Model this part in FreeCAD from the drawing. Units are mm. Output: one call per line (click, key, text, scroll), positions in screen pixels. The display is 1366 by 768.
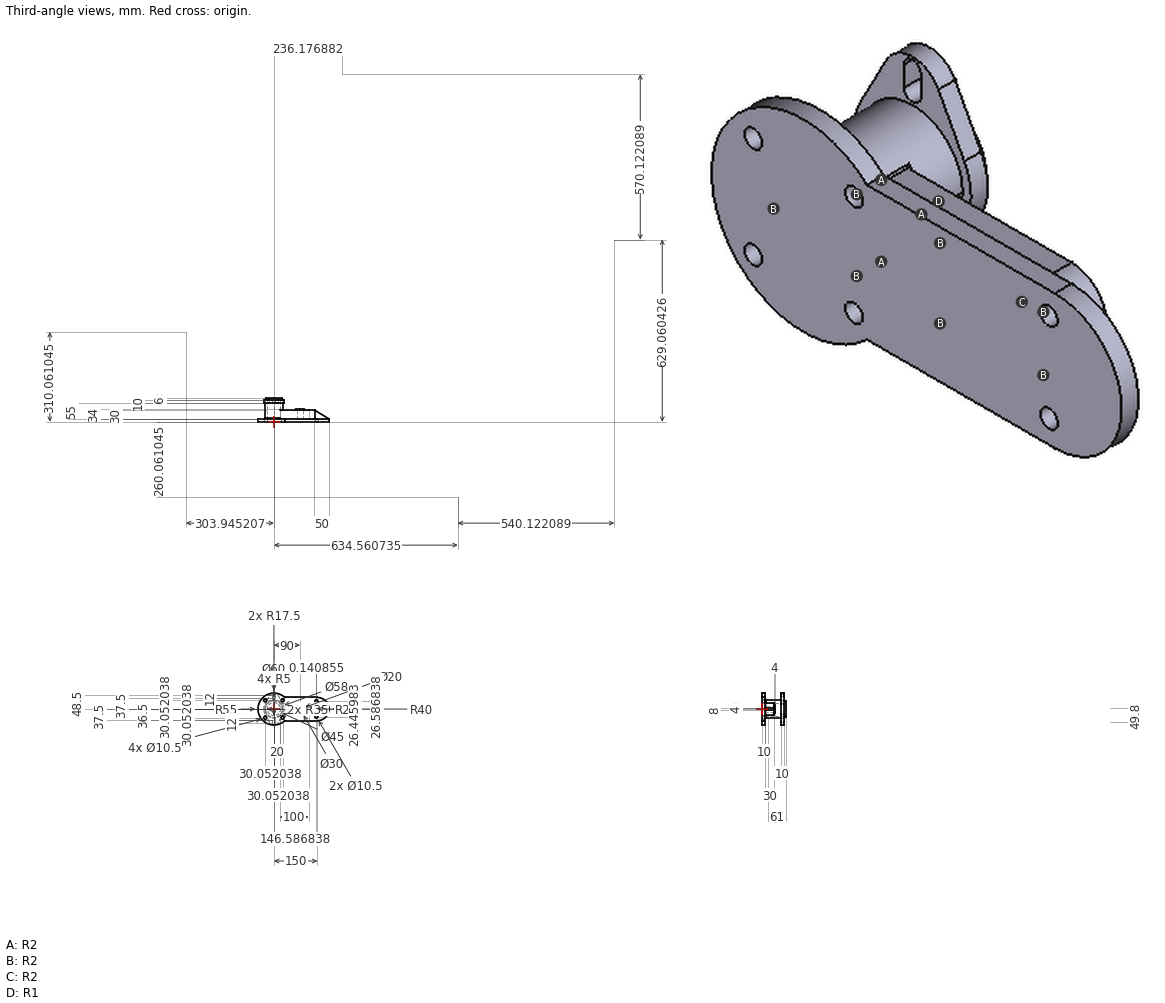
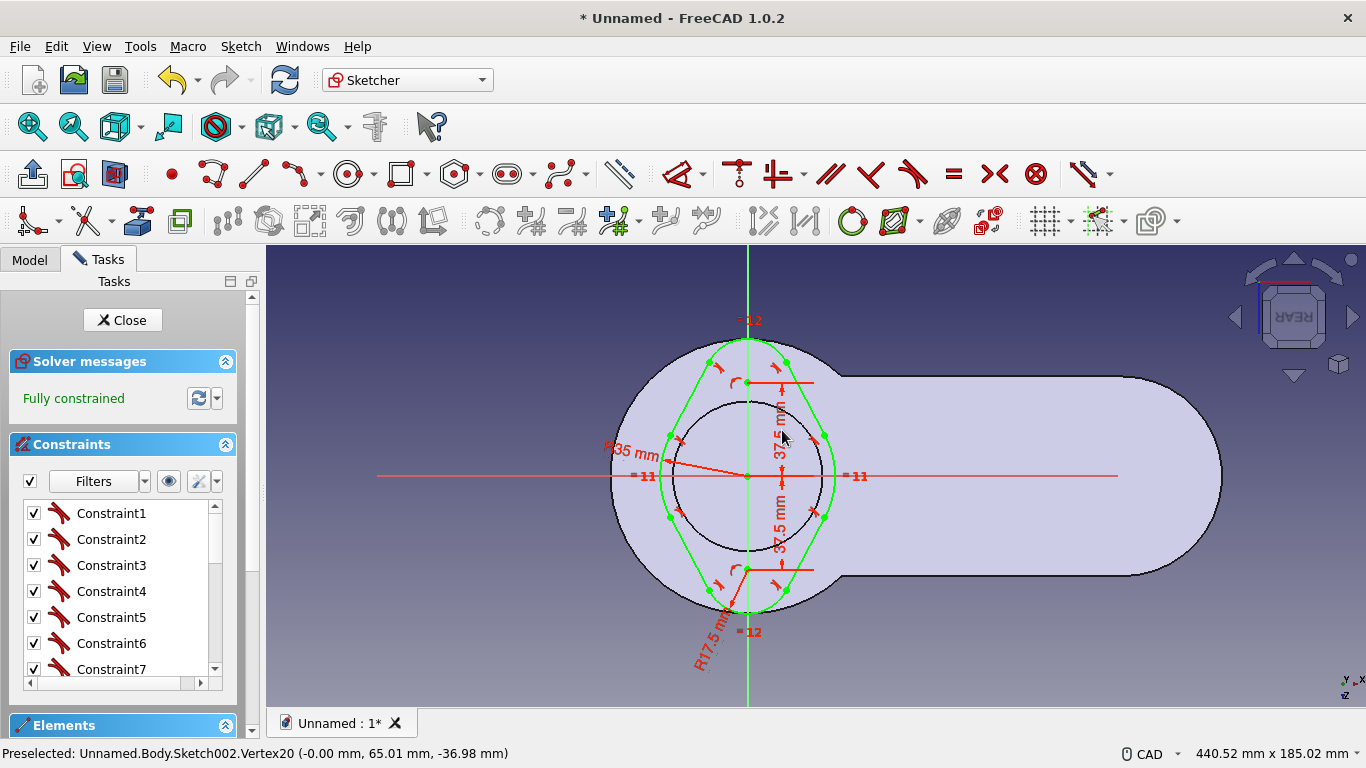
click(123, 320)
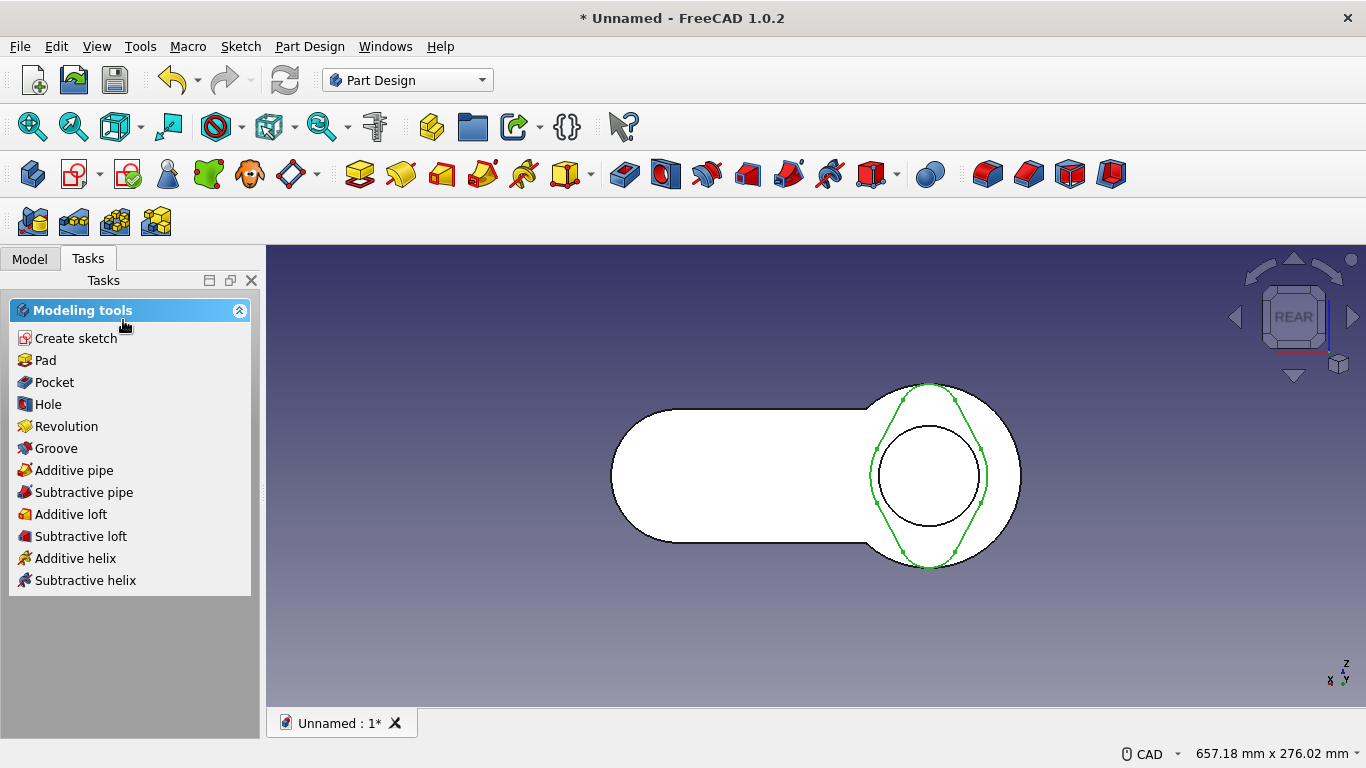
click(360, 174)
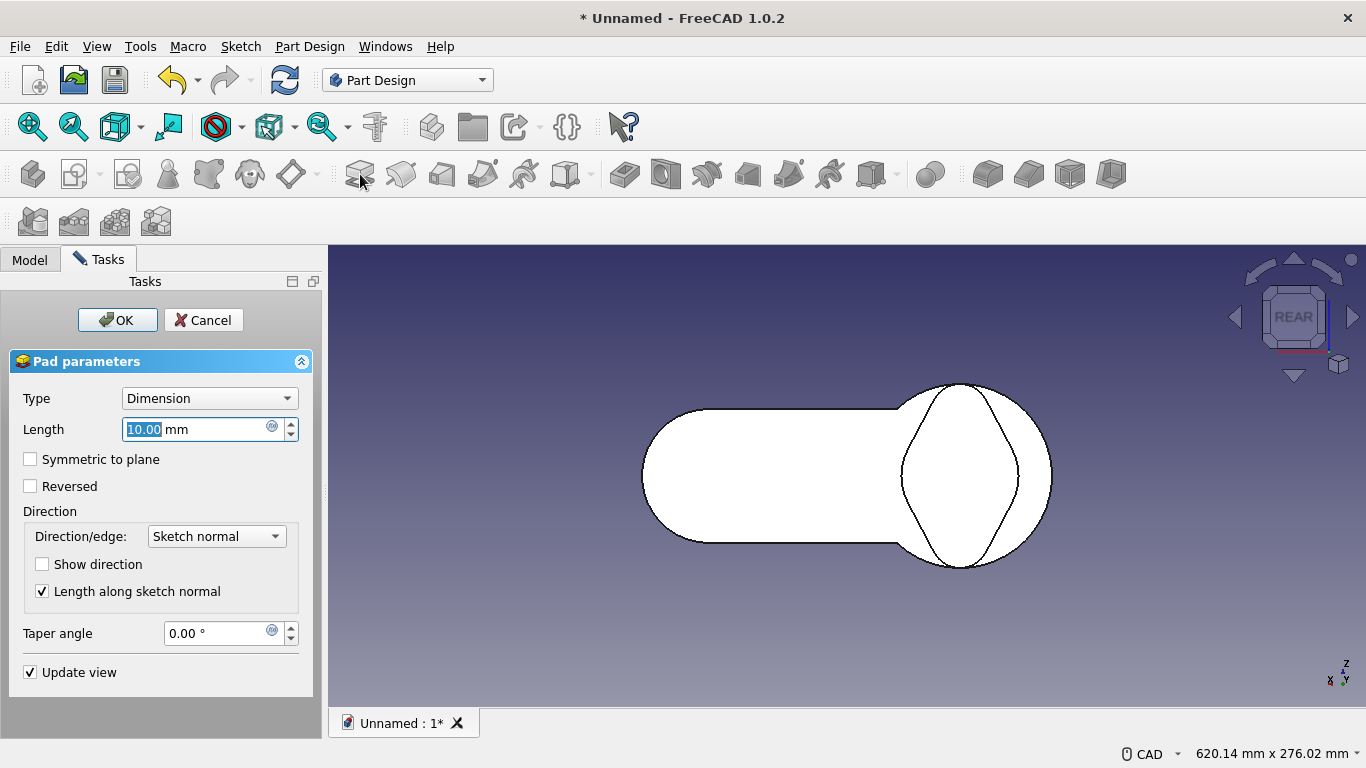
text(10)
key(Tab)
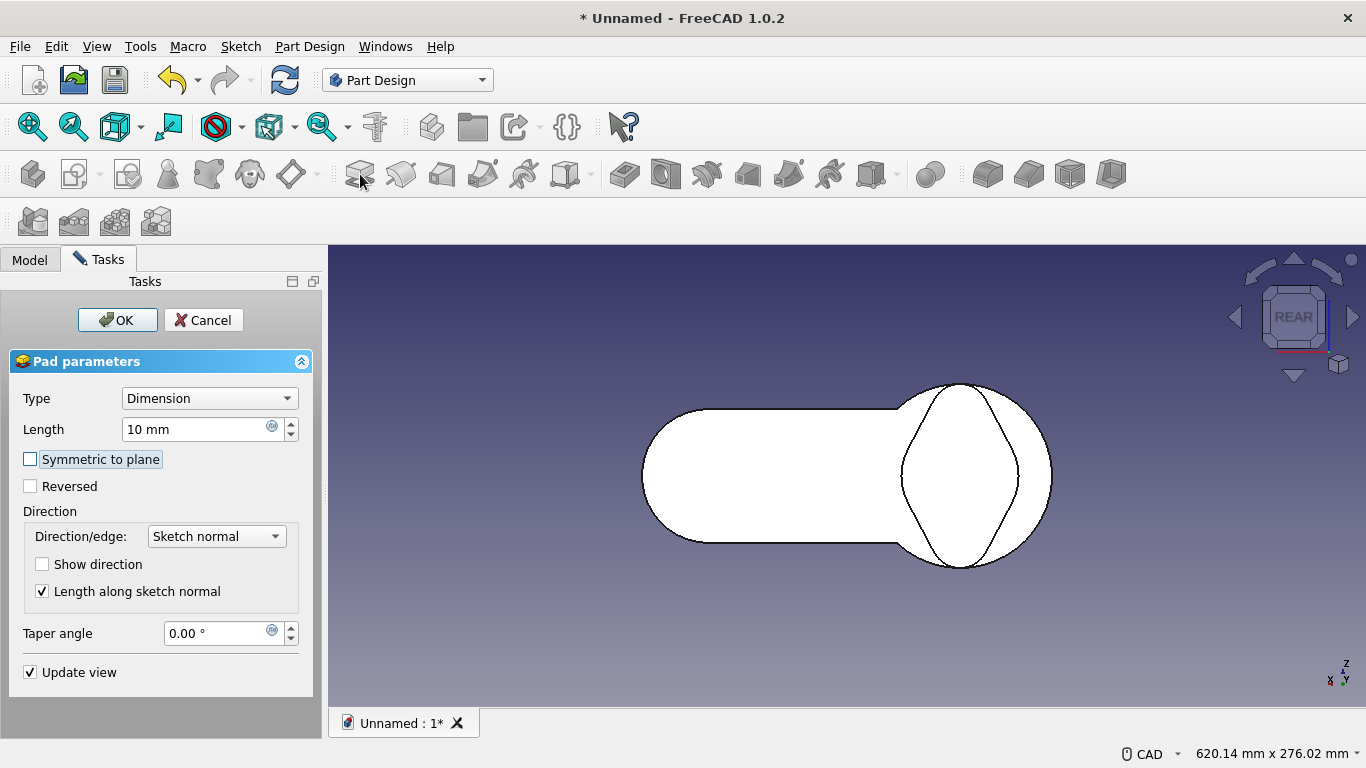
click(118, 320)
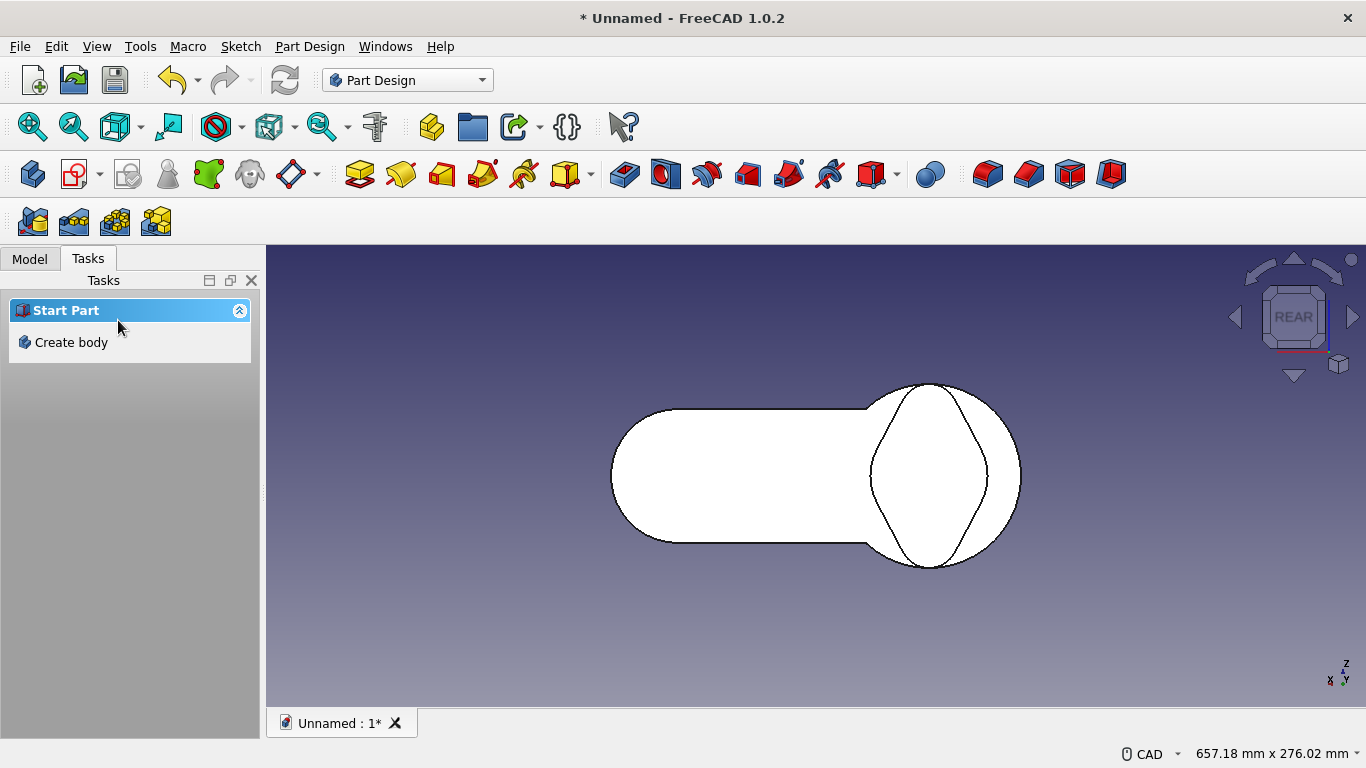
click(33, 128)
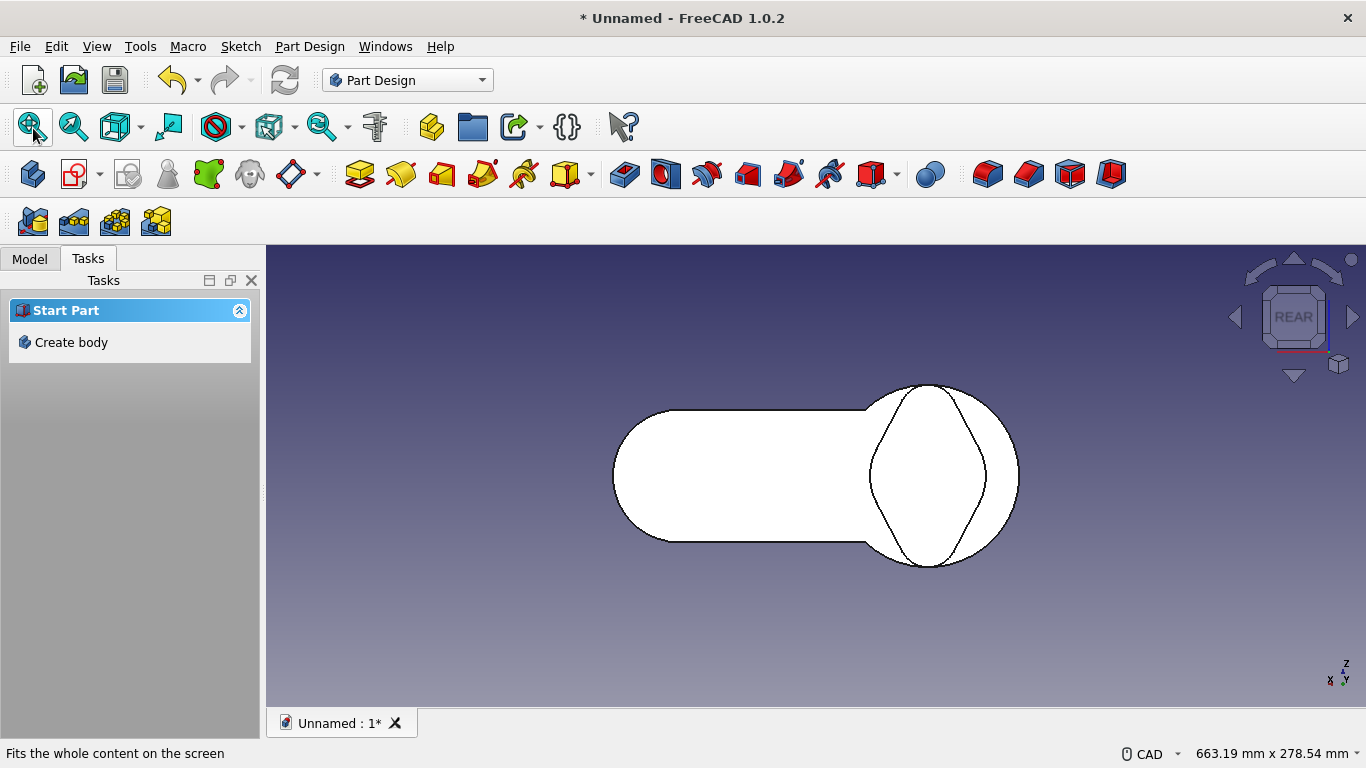
click(928, 475)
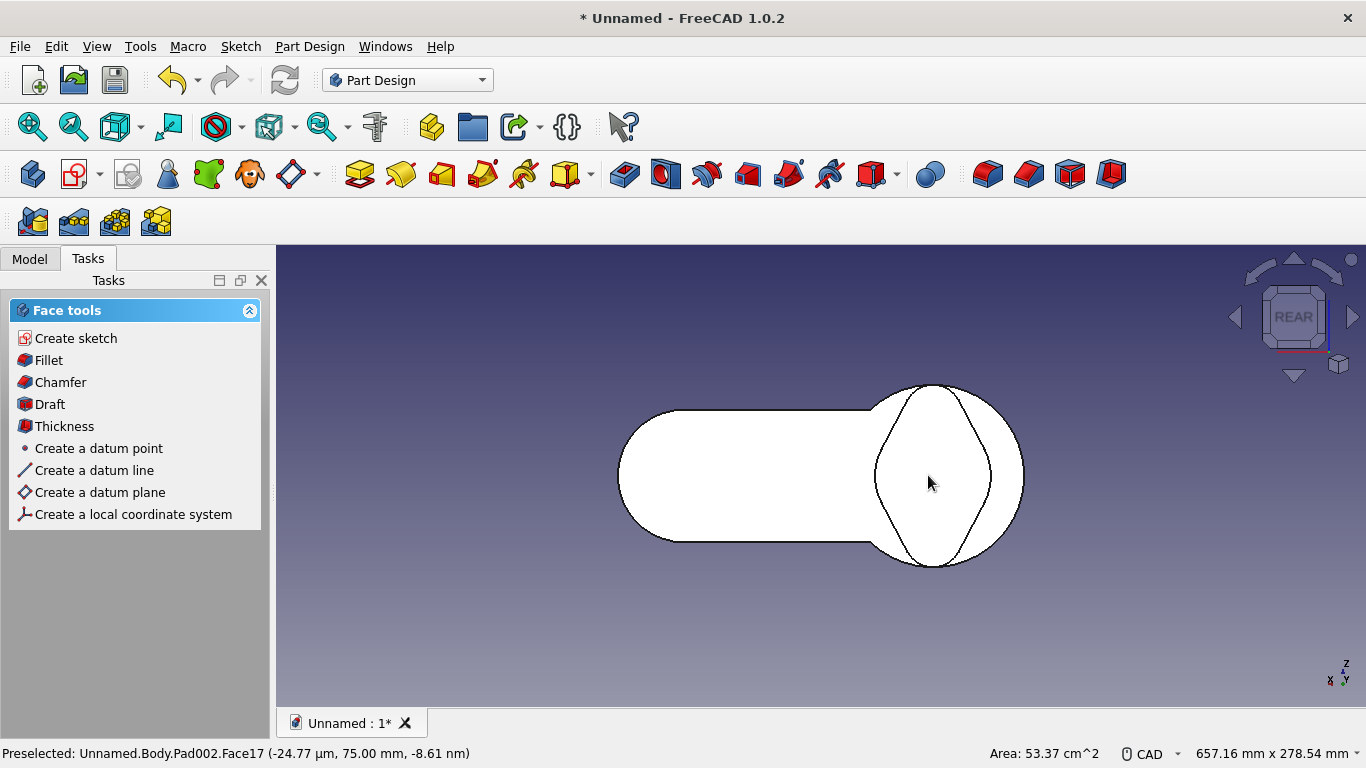
click(74, 174)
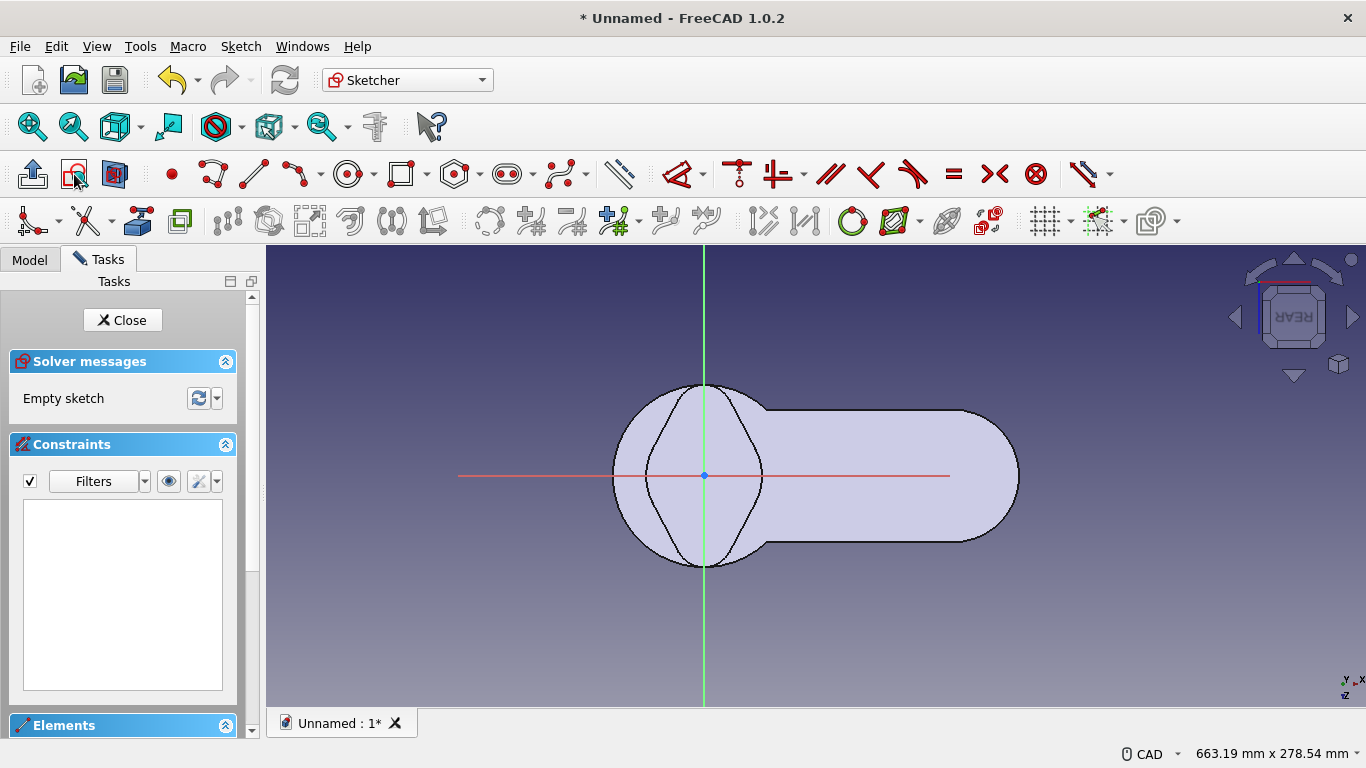
scroll(679, 476, up, 5)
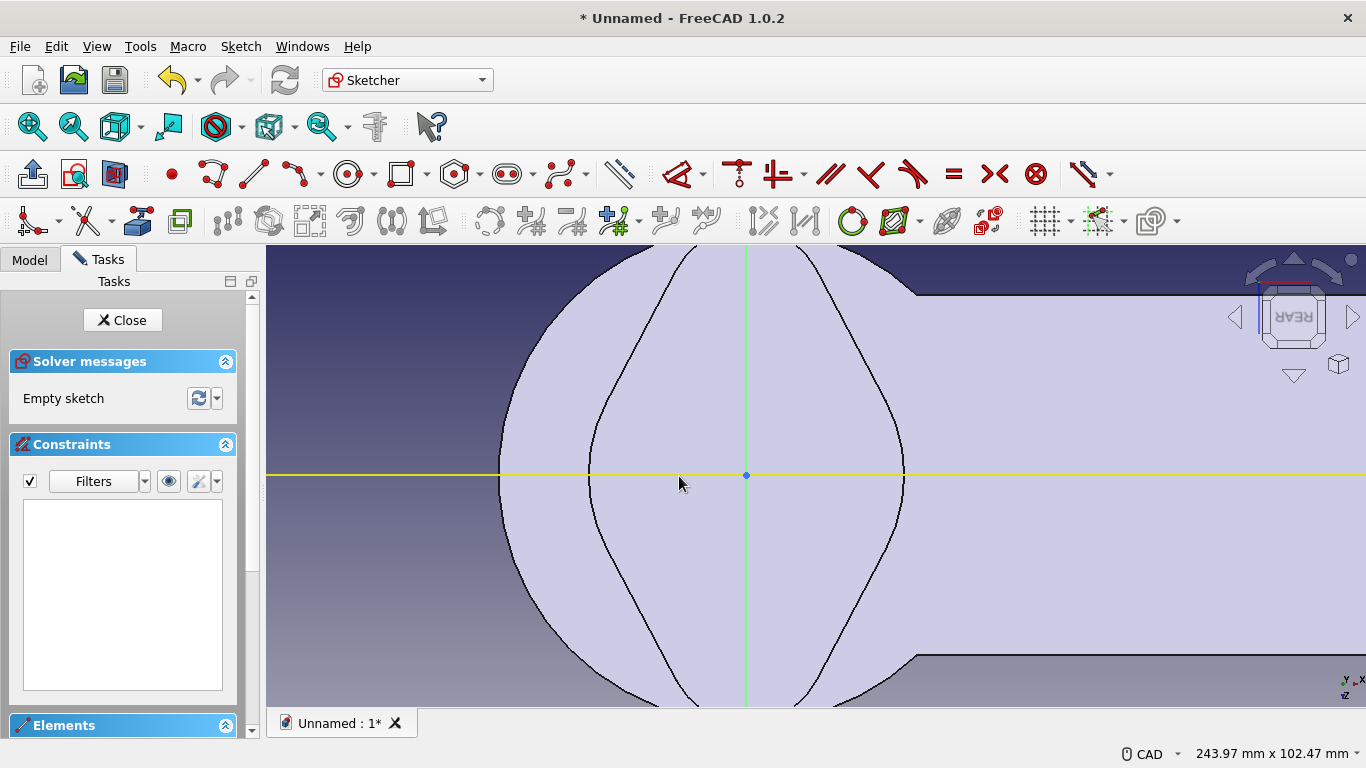
key(g)
key(c)